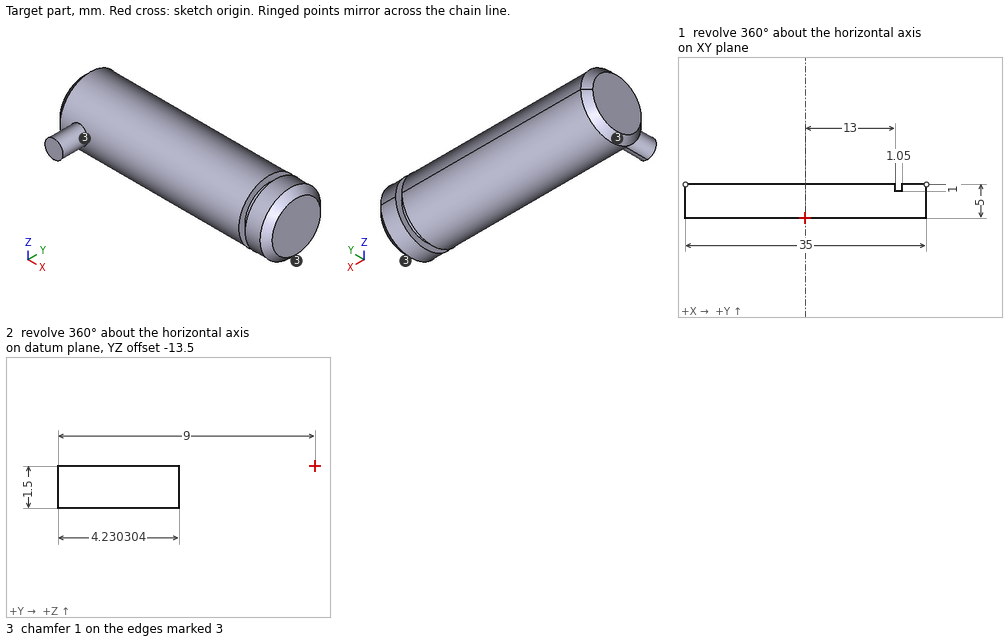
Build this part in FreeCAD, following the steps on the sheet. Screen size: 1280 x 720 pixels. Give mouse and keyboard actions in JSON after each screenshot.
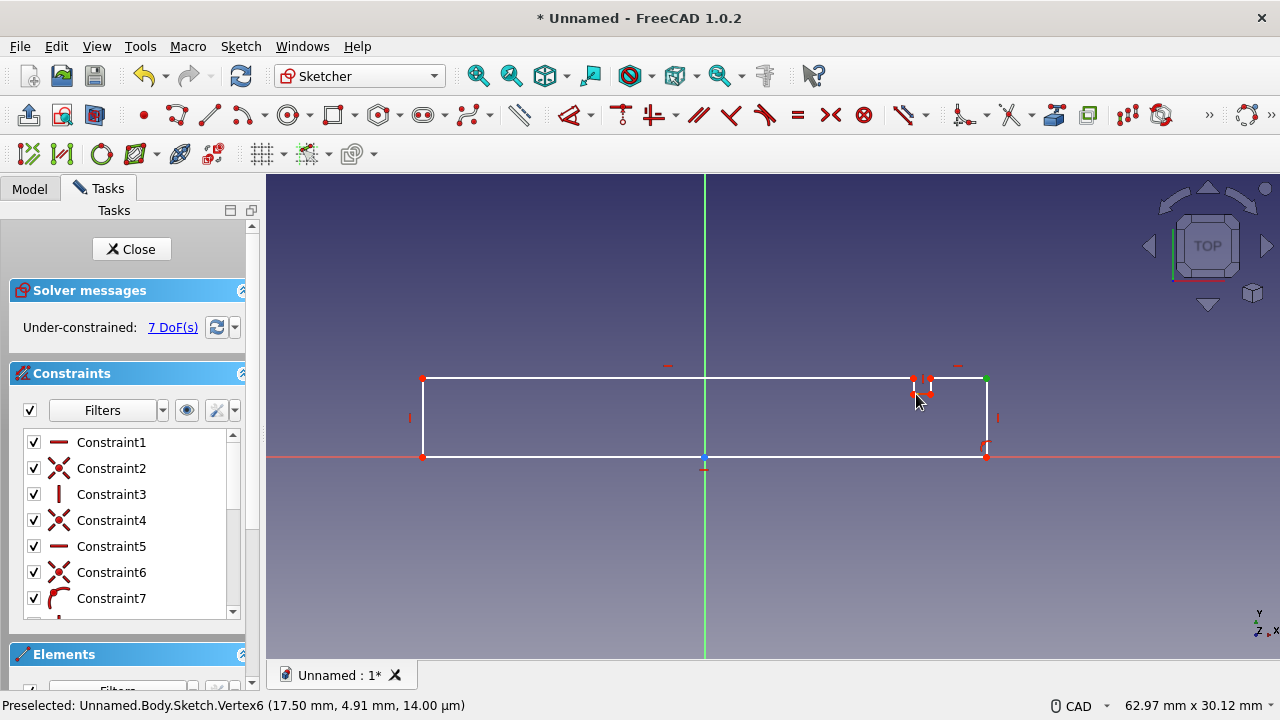
{"action": "left_click", "coordinate": [423, 378]}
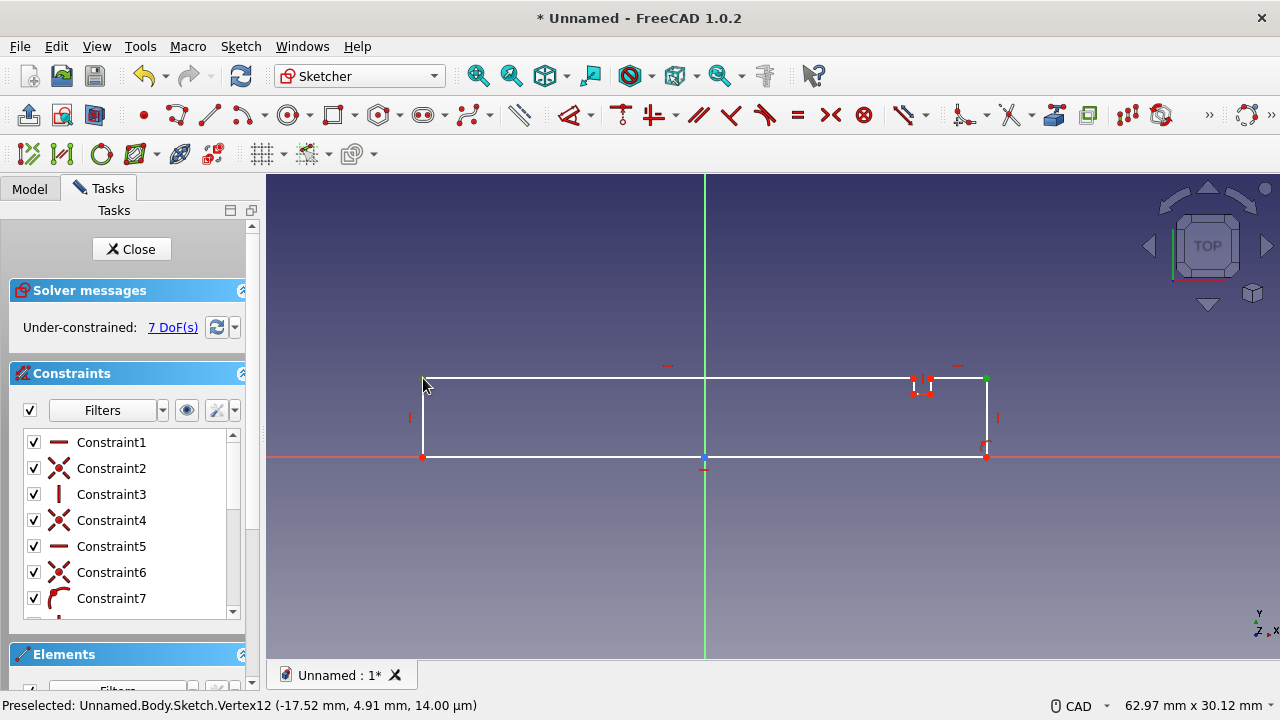
{"action": "left_click", "coordinate": [705, 600]}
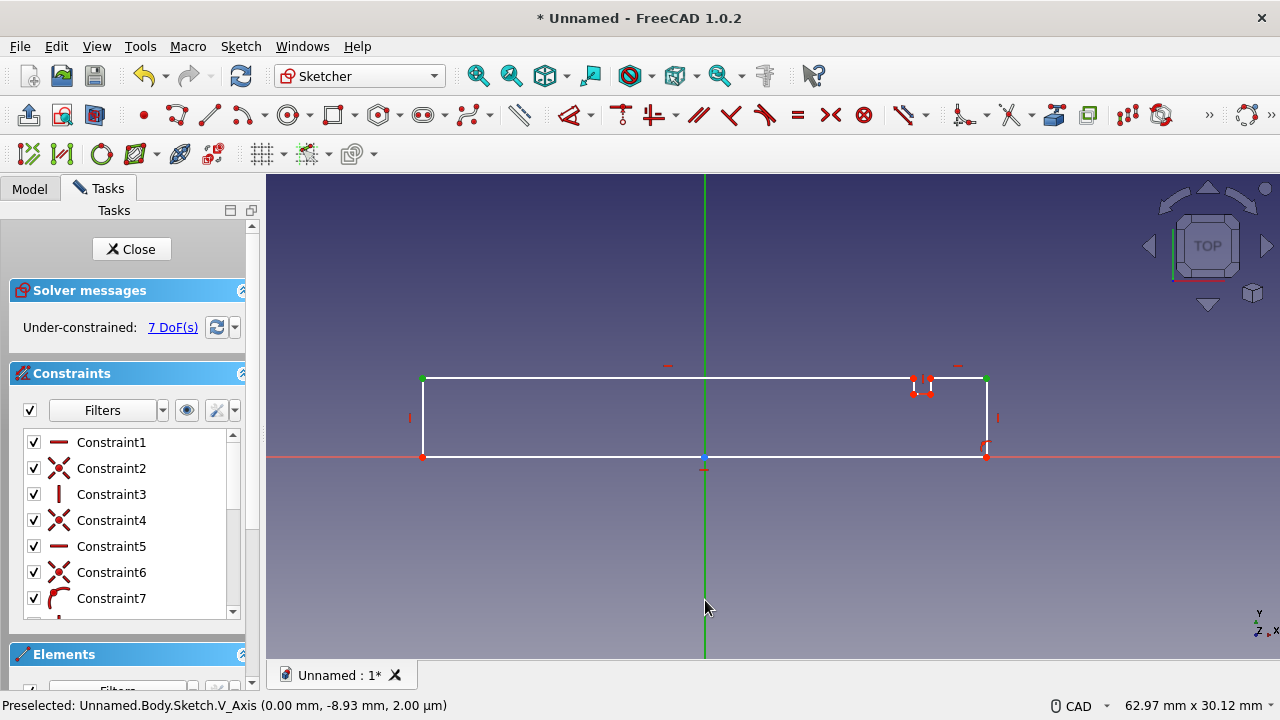
{"action": "key", "text": "s"}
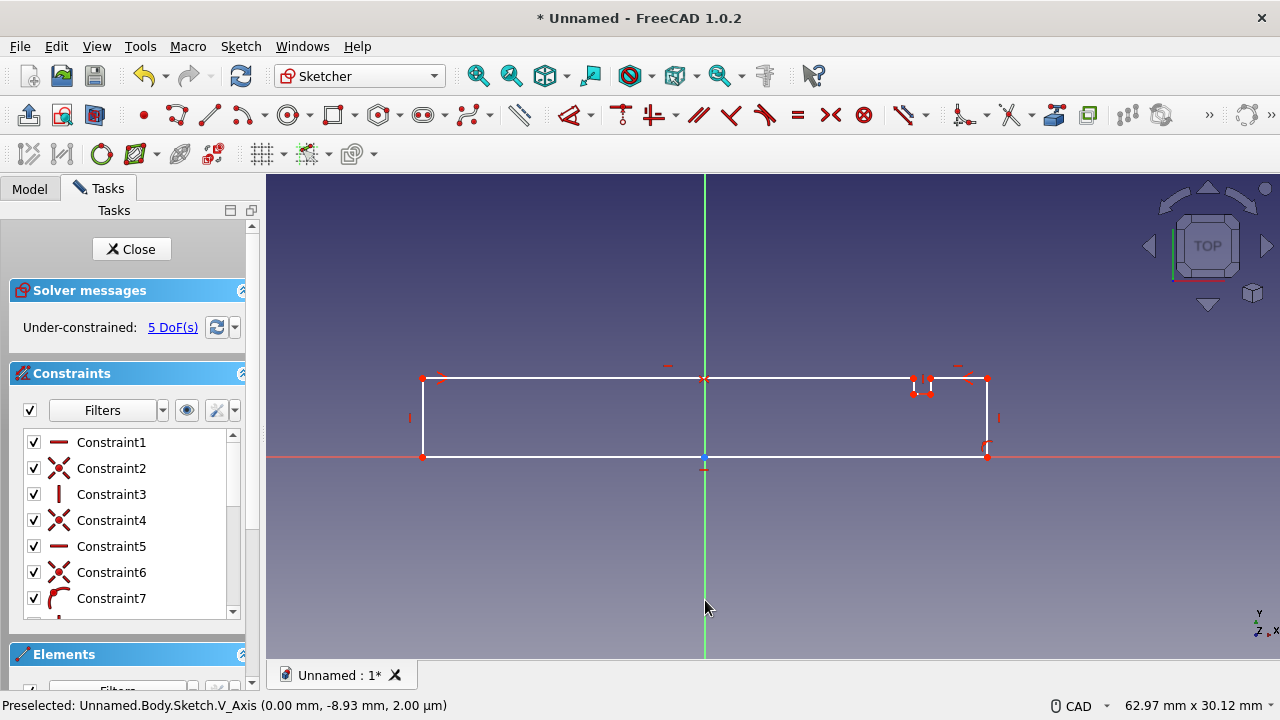
{"action": "scroll", "coordinate": [931, 386], "scroll_direction": "up", "scroll_amount": 5}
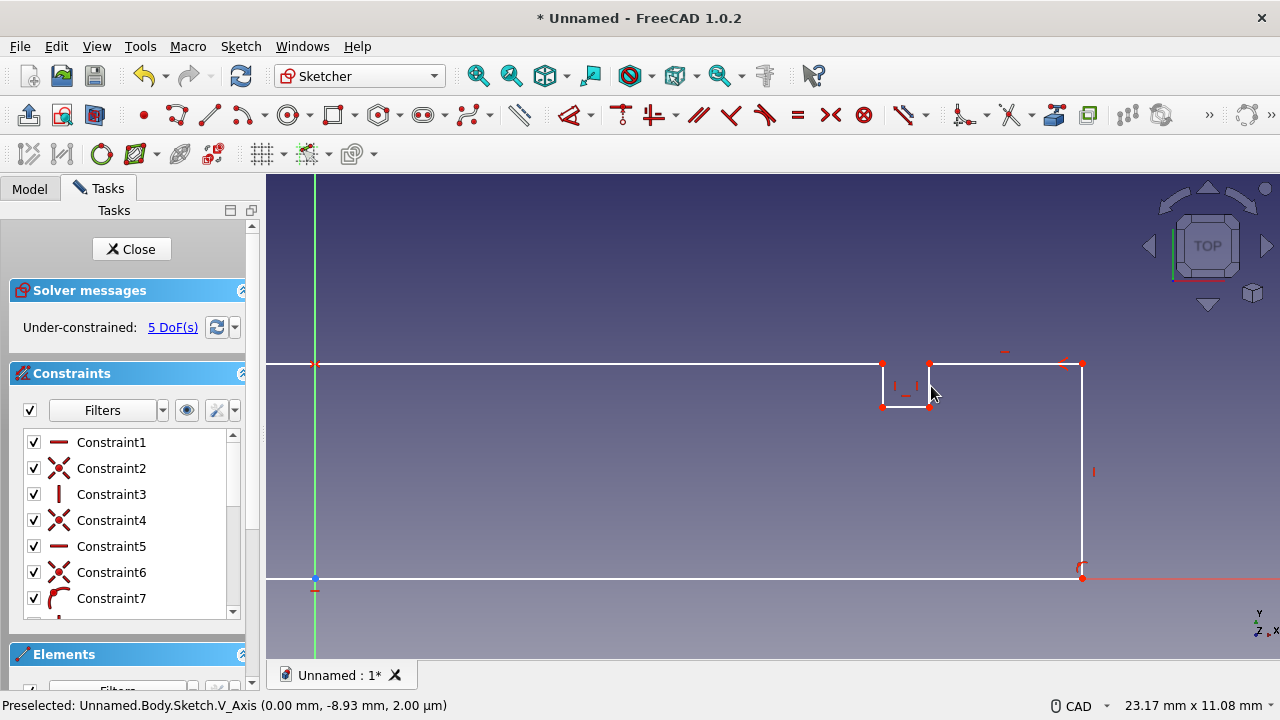
{"action": "left_click", "coordinate": [929, 386]}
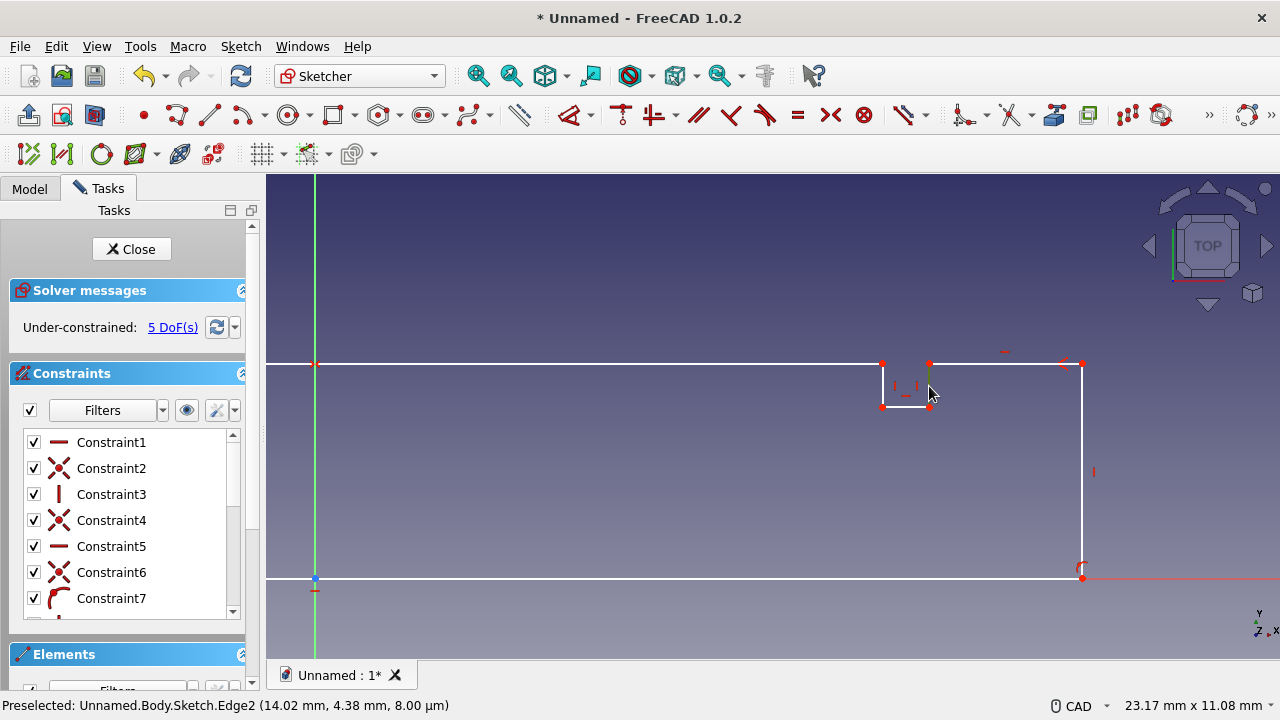
{"action": "key", "text": "i"}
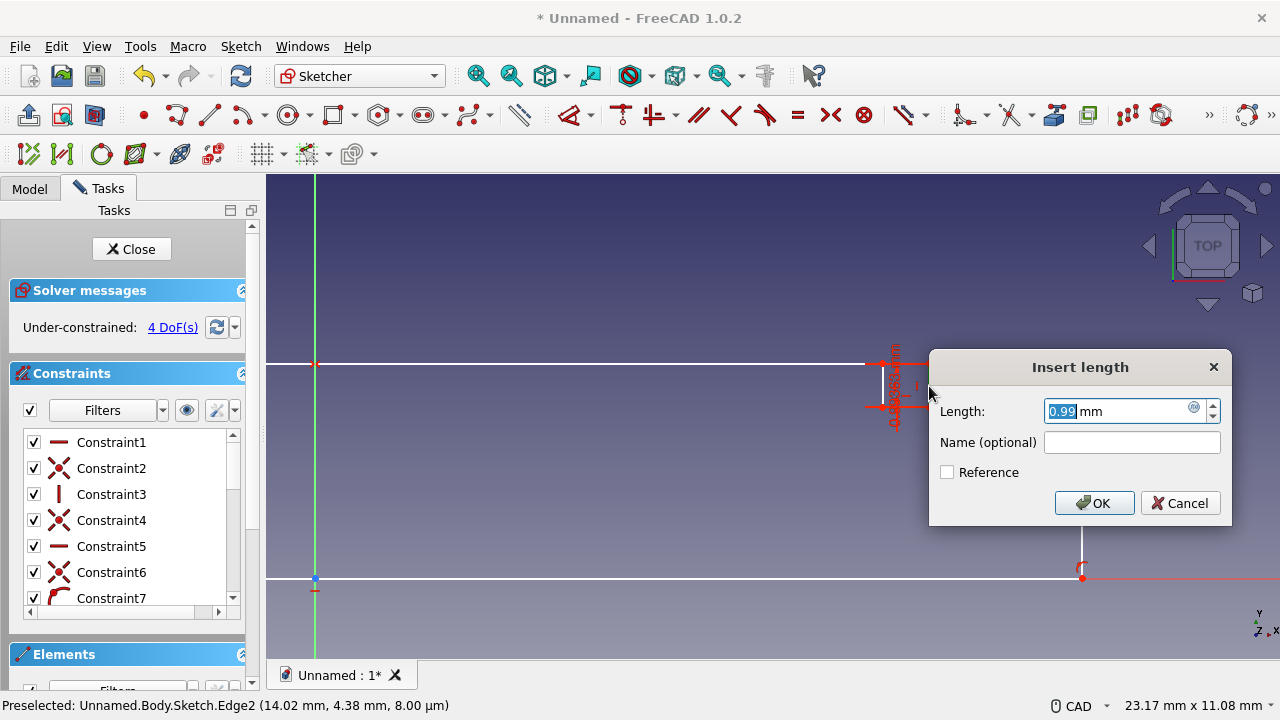
{"action": "type", "text": "1"}
{"action": "key", "text": "Return"}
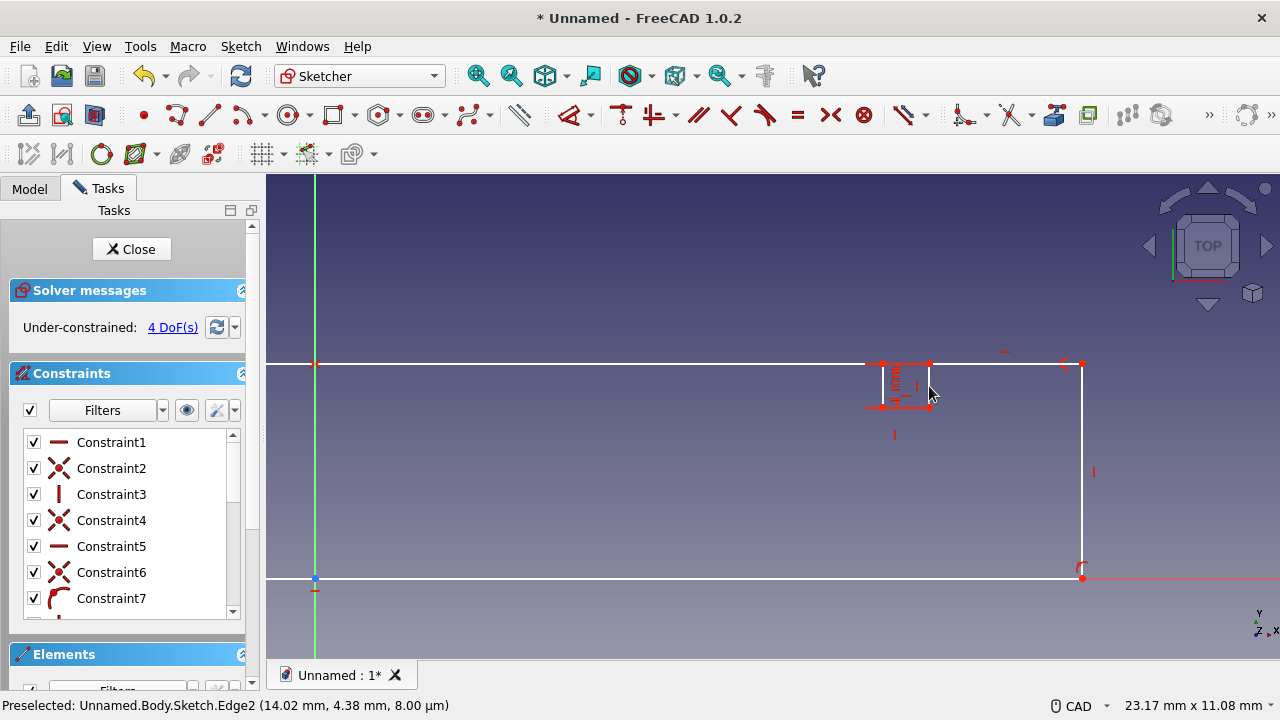
{"action": "left_click", "coordinate": [1082, 428]}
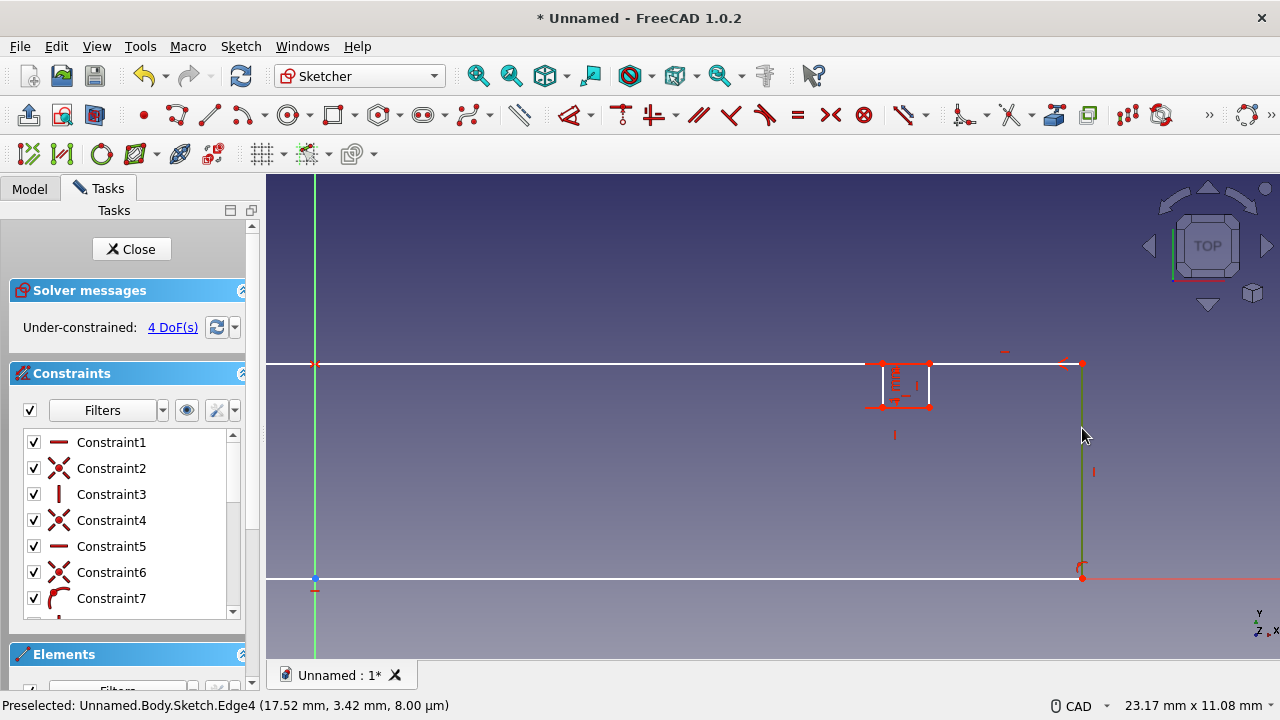
{"action": "left_click", "coordinate": [590, 116]}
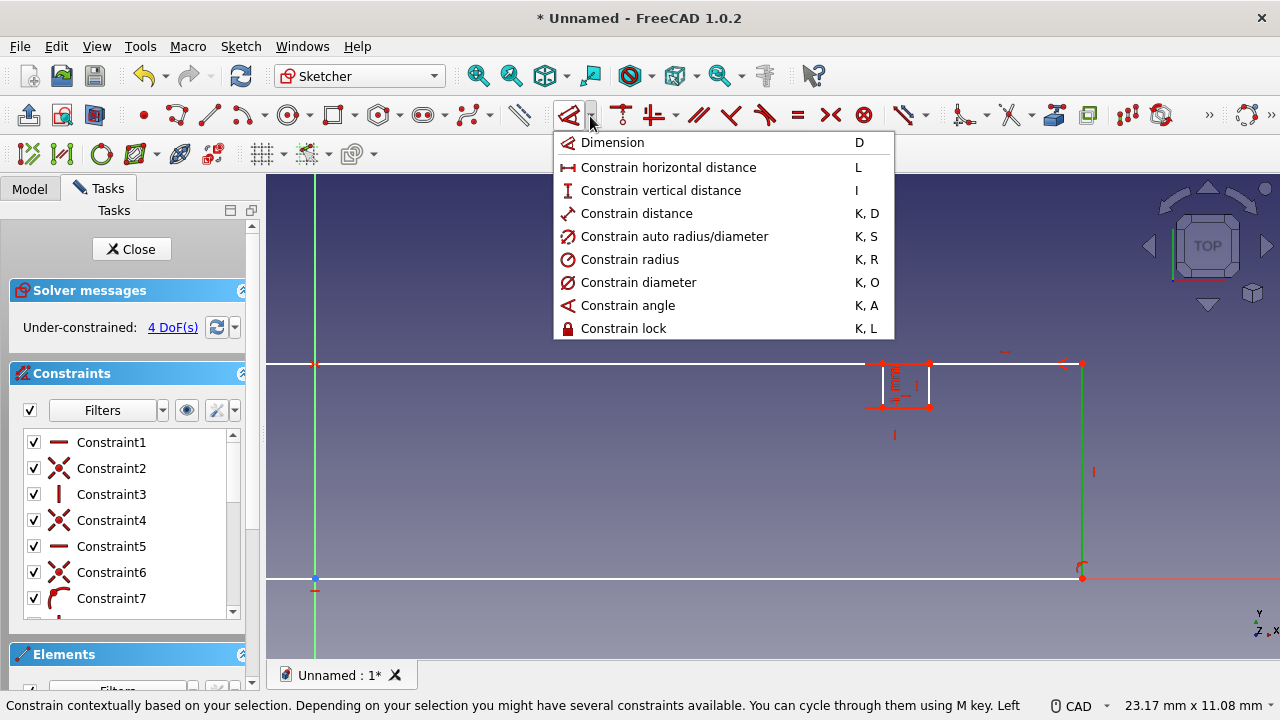
{"action": "left_click", "coordinate": [724, 190]}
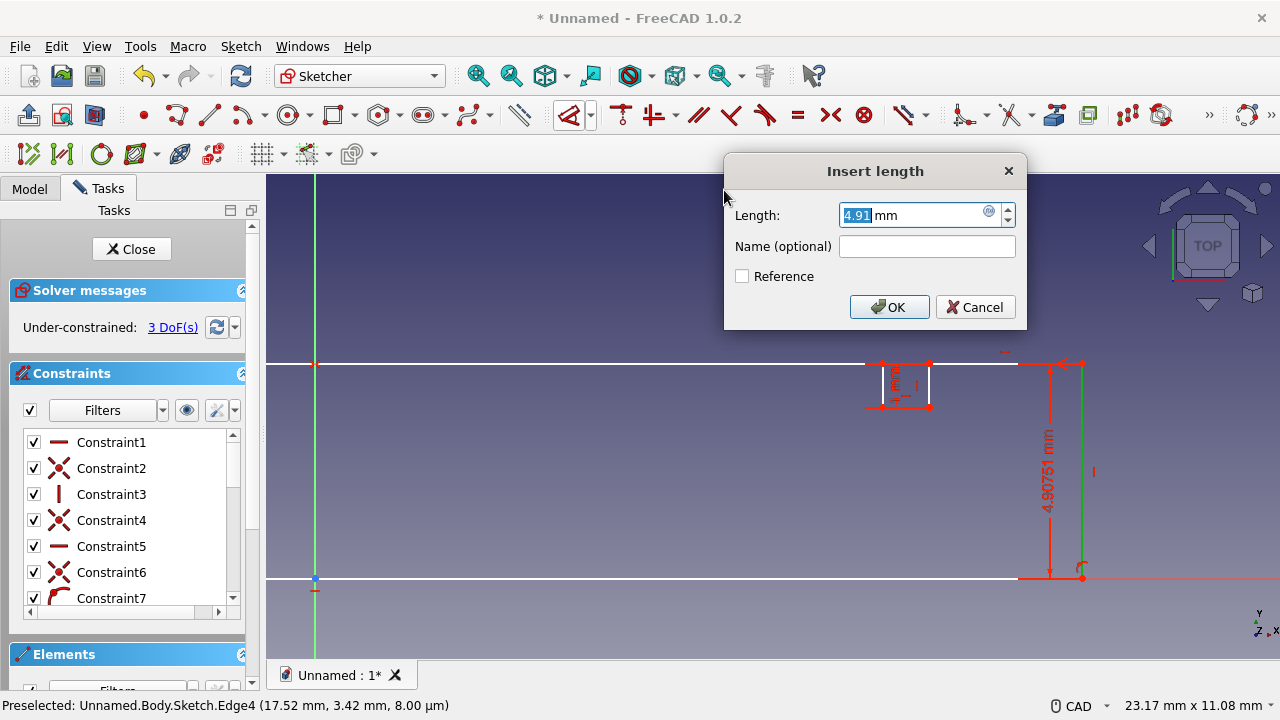
{"action": "type", "text": "5"}
{"action": "key", "text": "Return"}